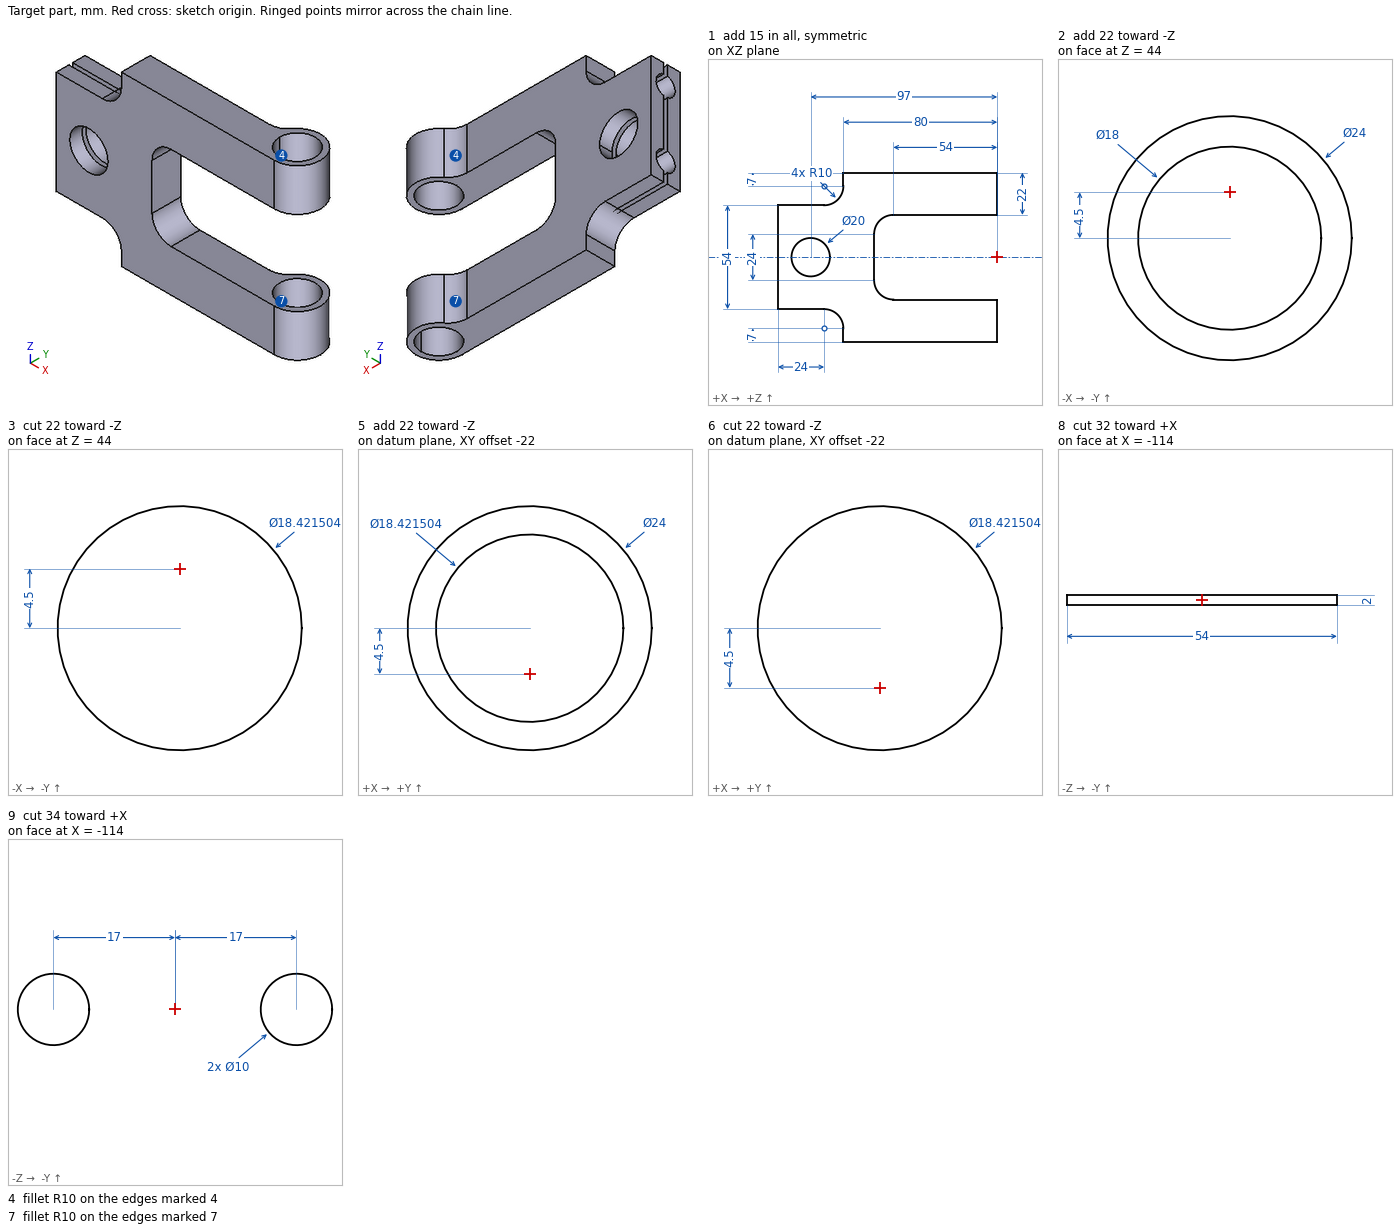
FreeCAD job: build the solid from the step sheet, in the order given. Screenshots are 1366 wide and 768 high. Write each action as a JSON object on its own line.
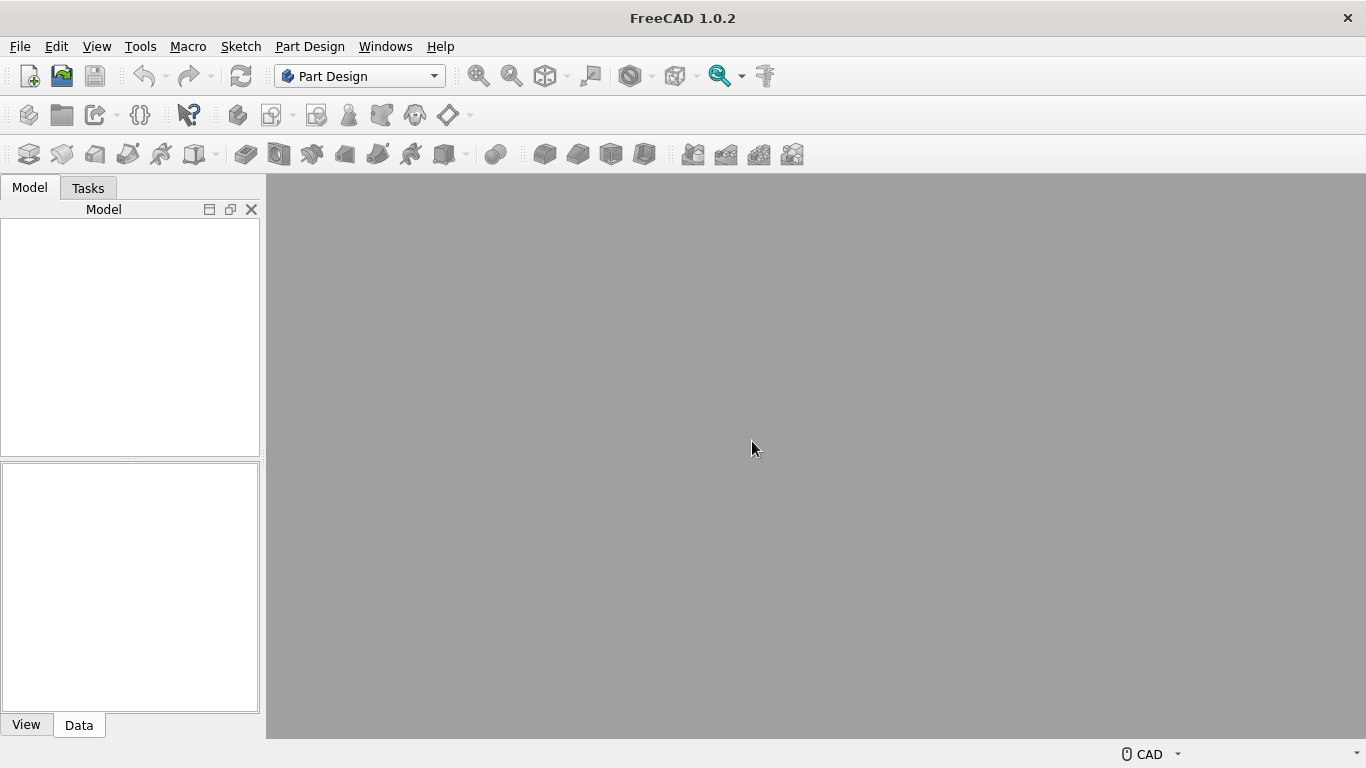
{"action": "left_click", "coordinate": [29, 76]}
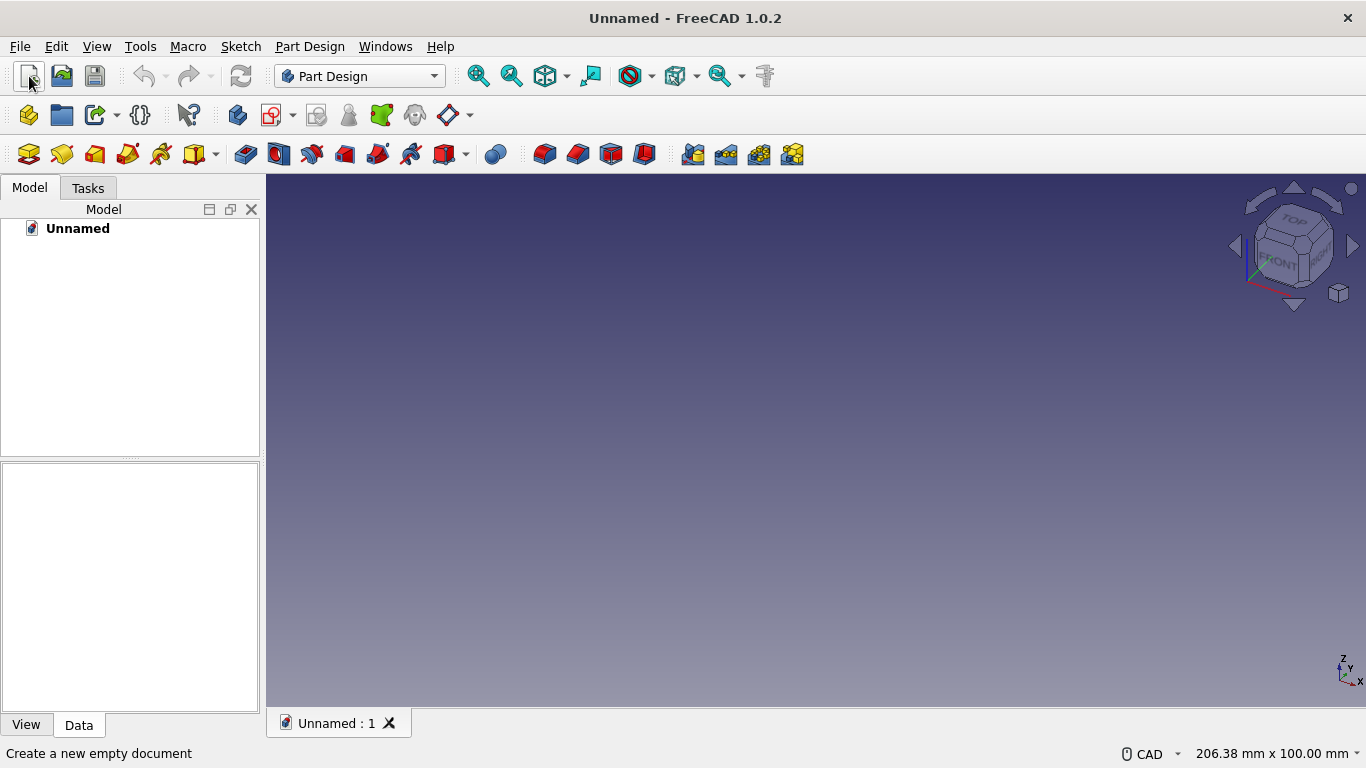
{"action": "left_click", "coordinate": [270, 116]}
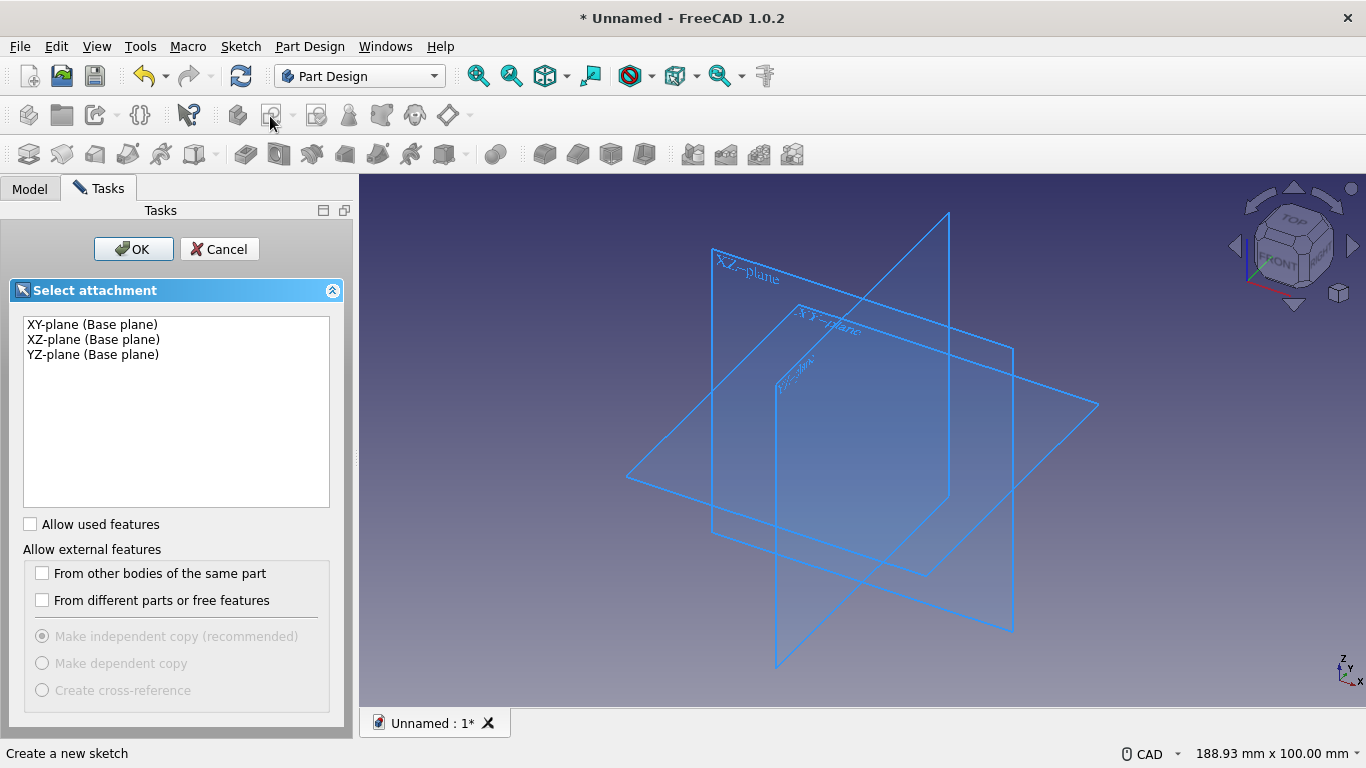
{"action": "left_click", "coordinate": [84, 340]}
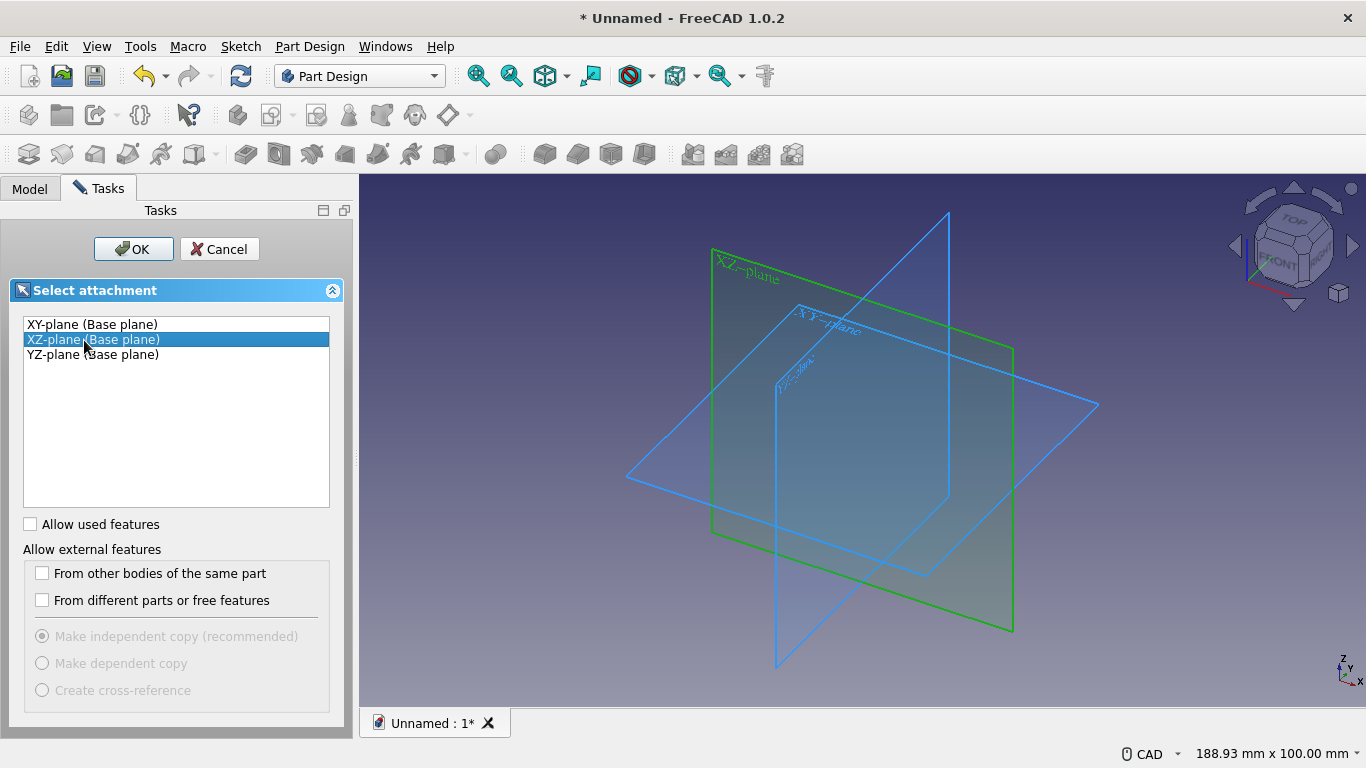
{"action": "left_click", "coordinate": [134, 249]}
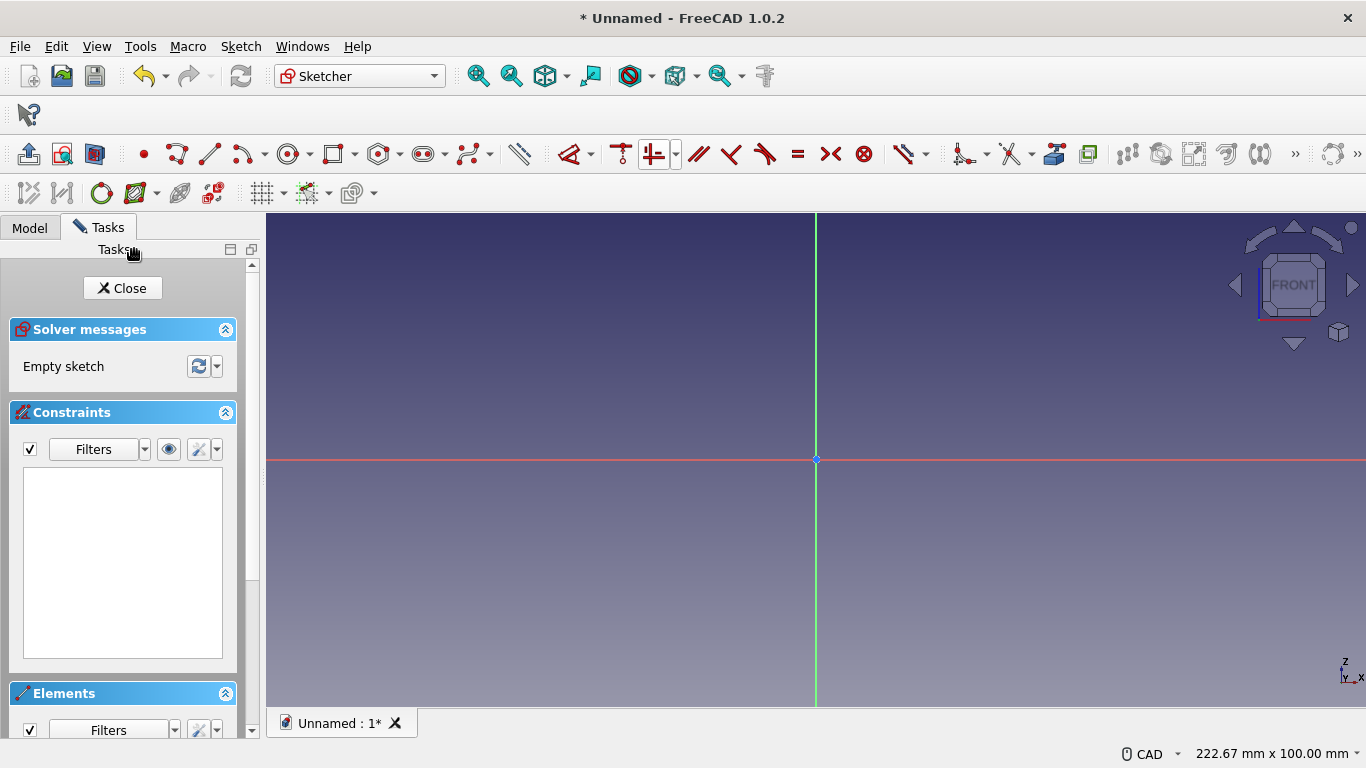
{"action": "scroll", "coordinate": [1181, 460], "scroll_direction": "down", "scroll_amount": 2}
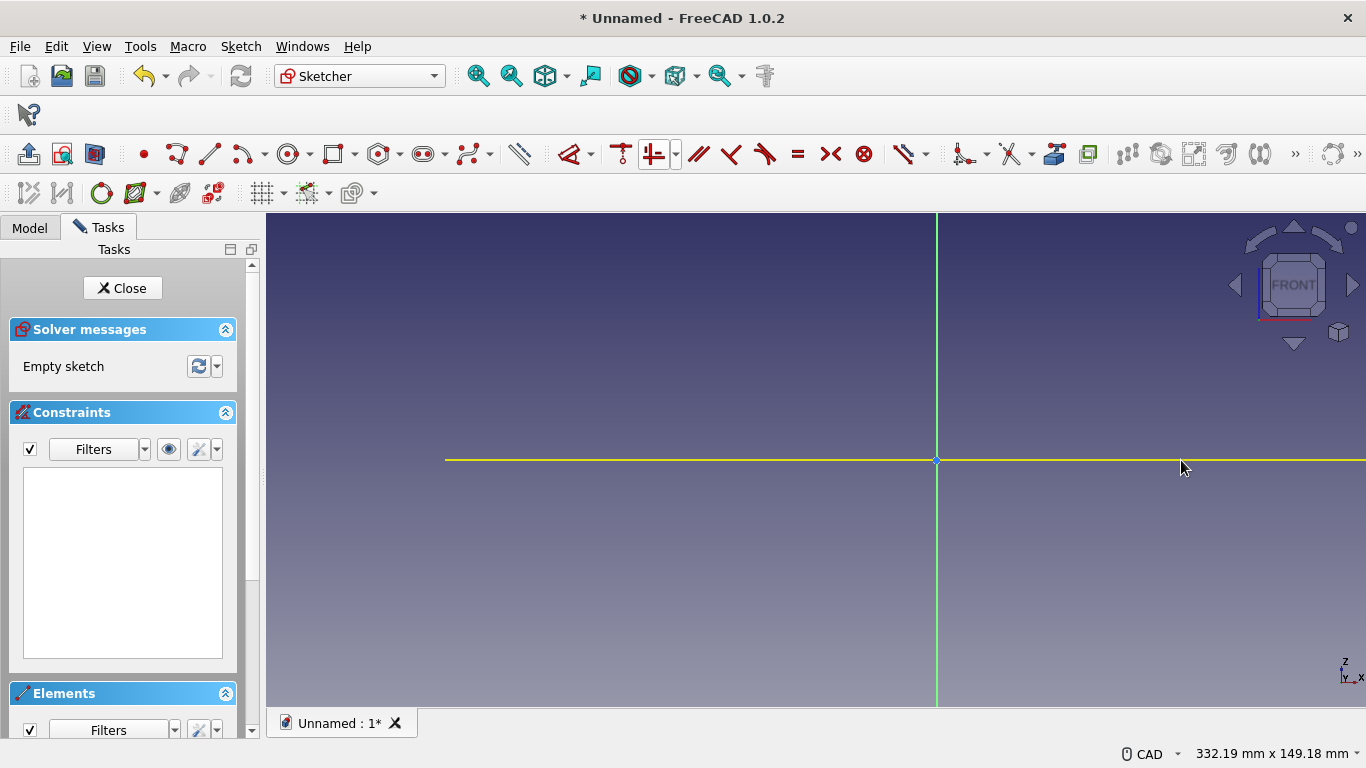
{"action": "left_click", "coordinate": [177, 154]}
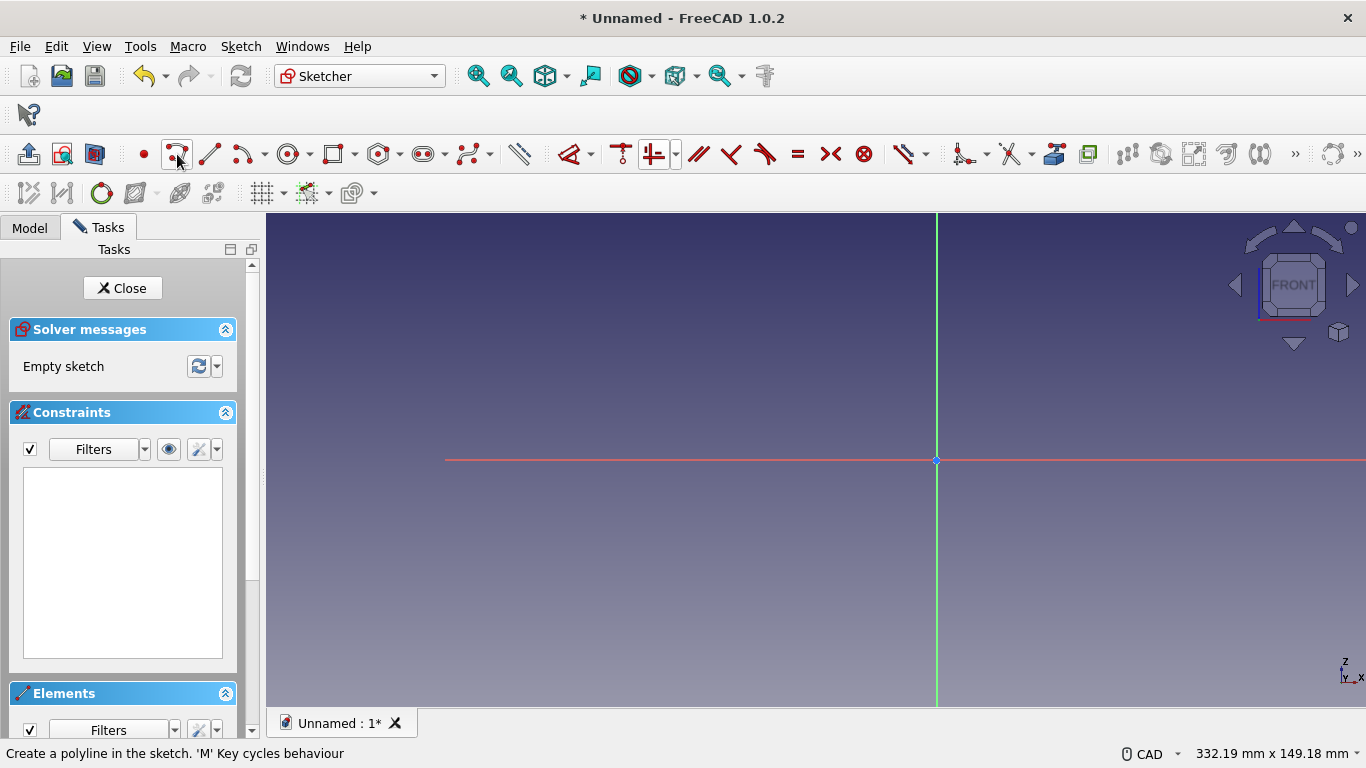
{"action": "left_click", "coordinate": [639, 550]}
{"action": "left_click", "coordinate": [559, 550]}
{"action": "left_click", "coordinate": [559, 371]}
{"action": "left_click", "coordinate": [639, 371]}
{"action": "right_click", "coordinate": [639, 371]}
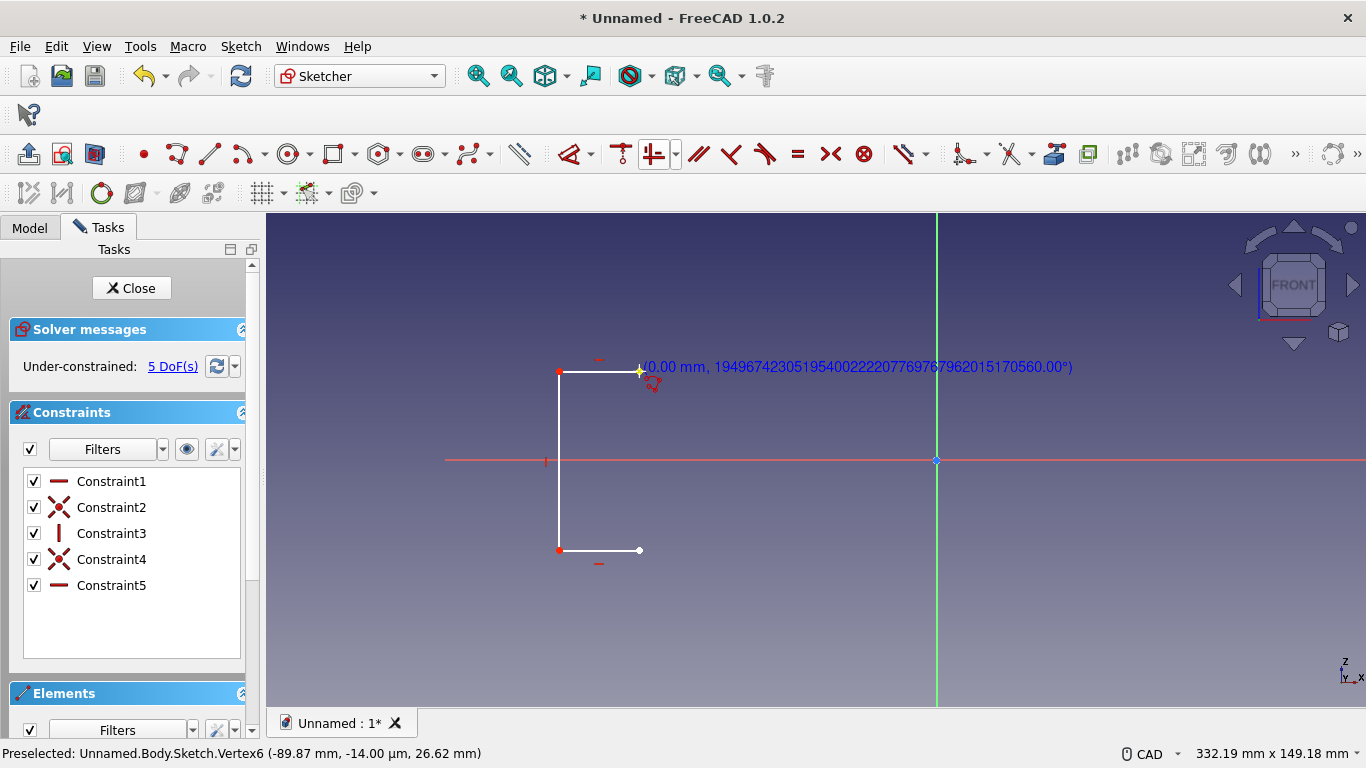
{"action": "left_click", "coordinate": [672, 338]}
{"action": "left_click", "coordinate": [672, 314]}
{"action": "left_click", "coordinate": [937, 314]}
{"action": "left_click", "coordinate": [928, 387]}
{"action": "left_click", "coordinate": [758, 387]}
{"action": "right_click", "coordinate": [758, 387]}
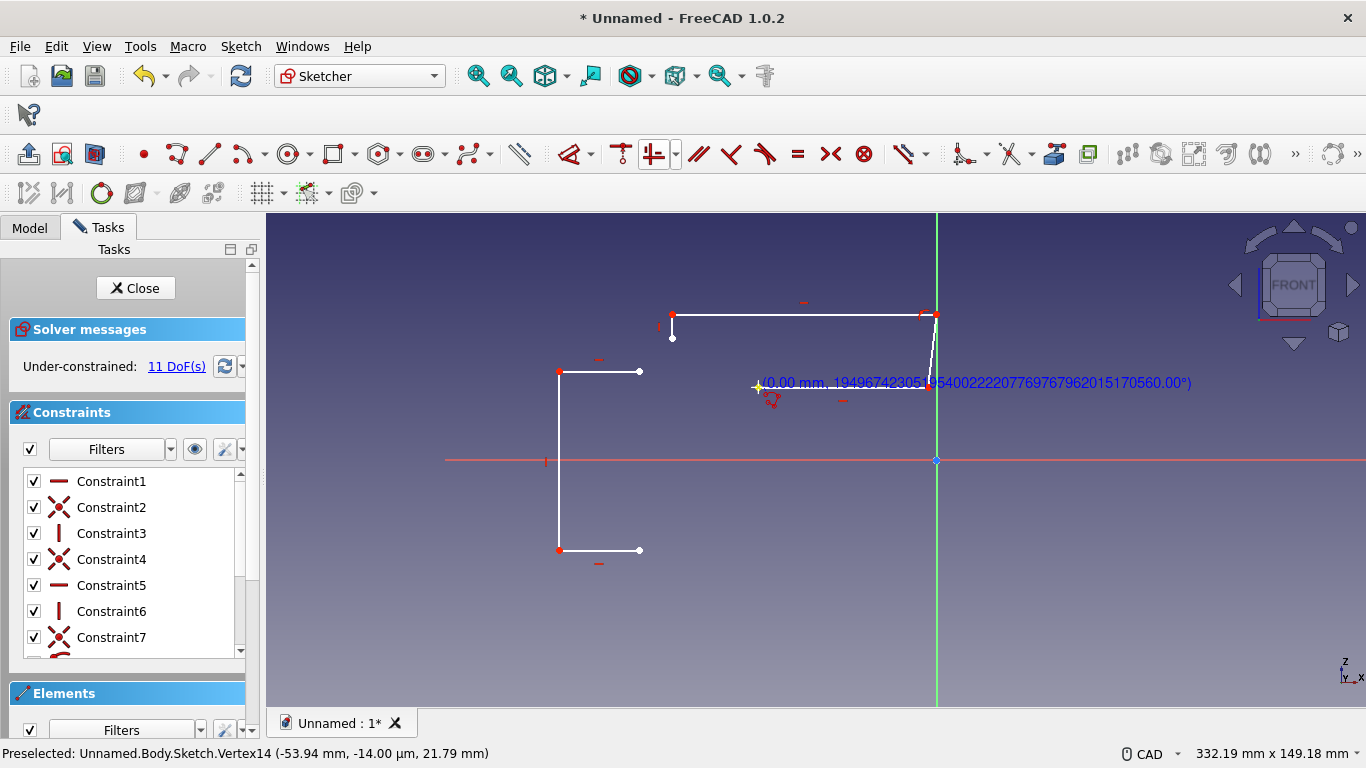
{"action": "left_click", "coordinate": [210, 154]}